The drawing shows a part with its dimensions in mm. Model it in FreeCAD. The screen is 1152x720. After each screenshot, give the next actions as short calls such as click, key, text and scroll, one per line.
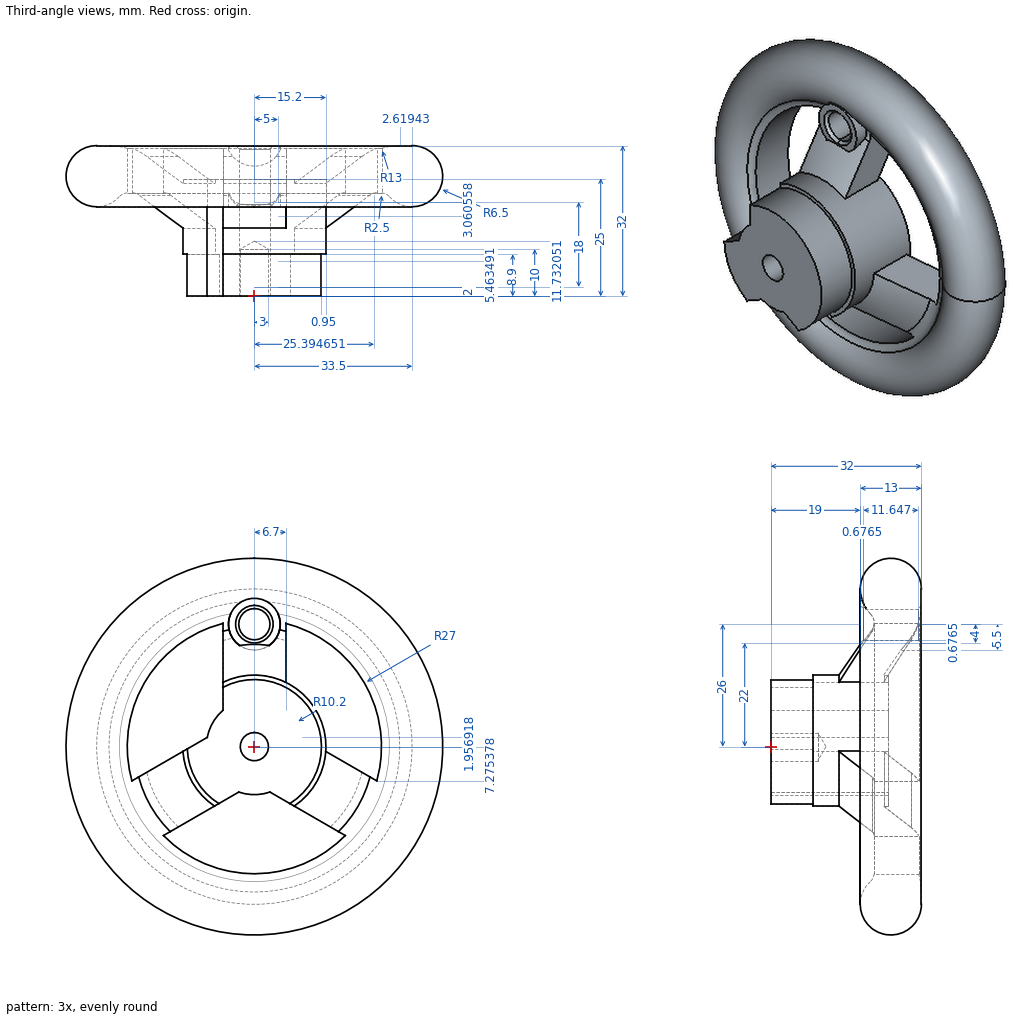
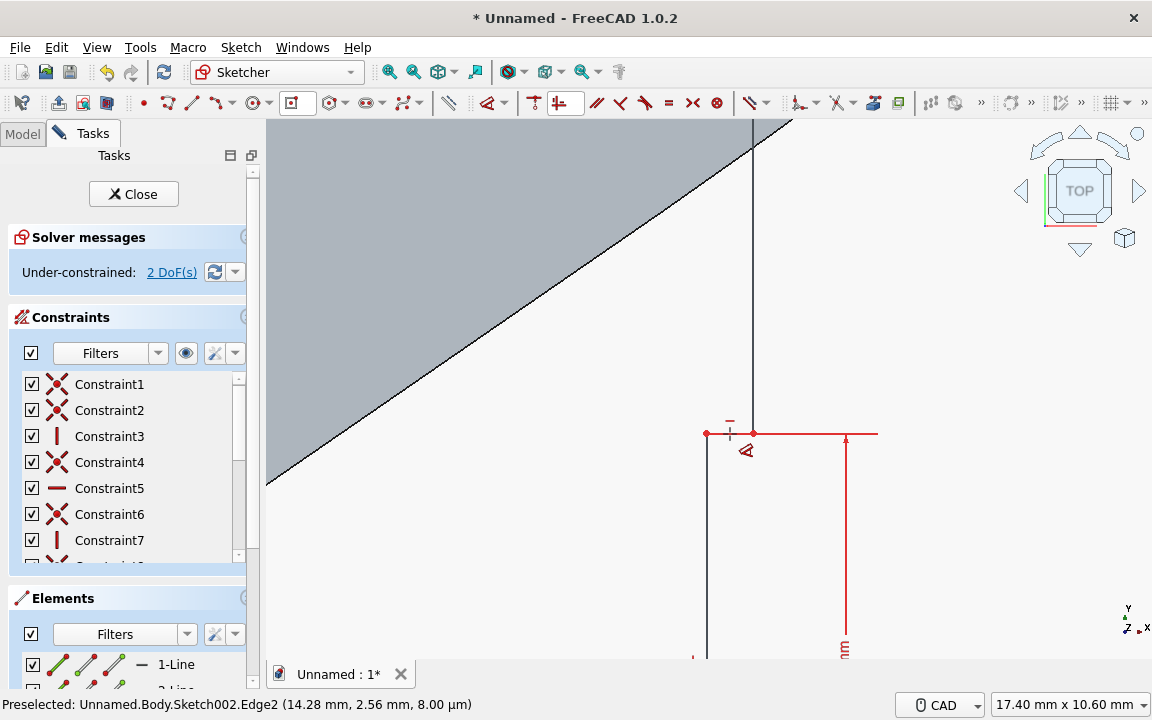
click(730, 434)
click(730, 468)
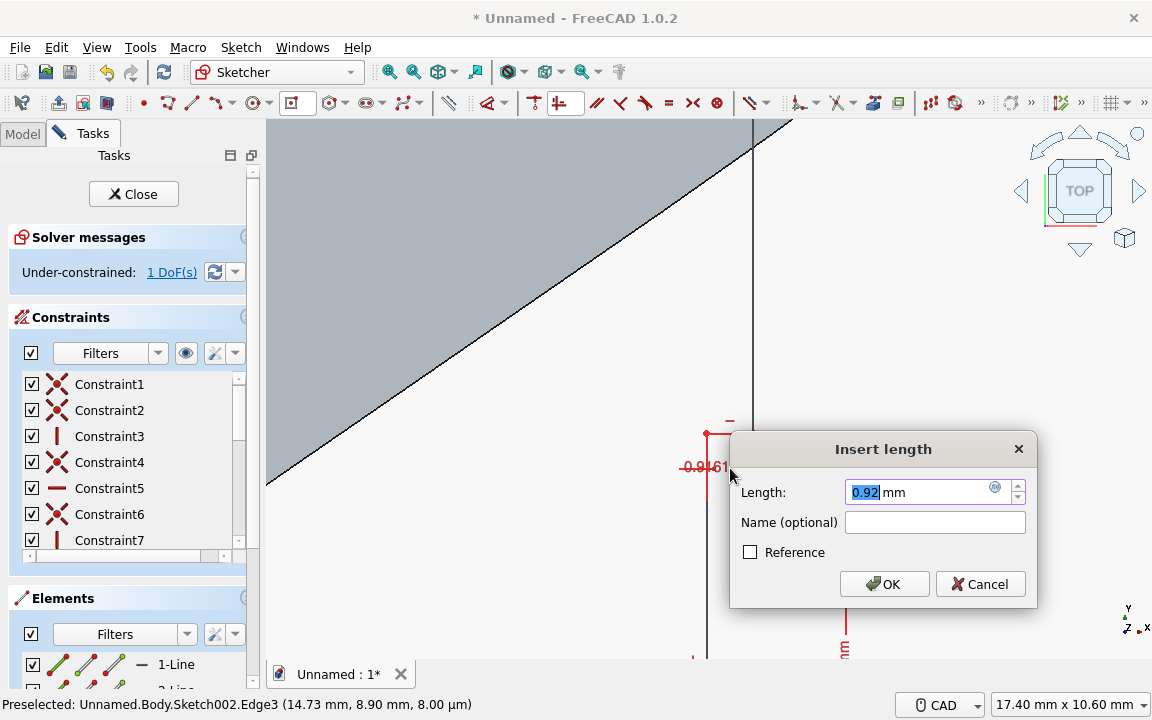
text(0.95)
key(Return)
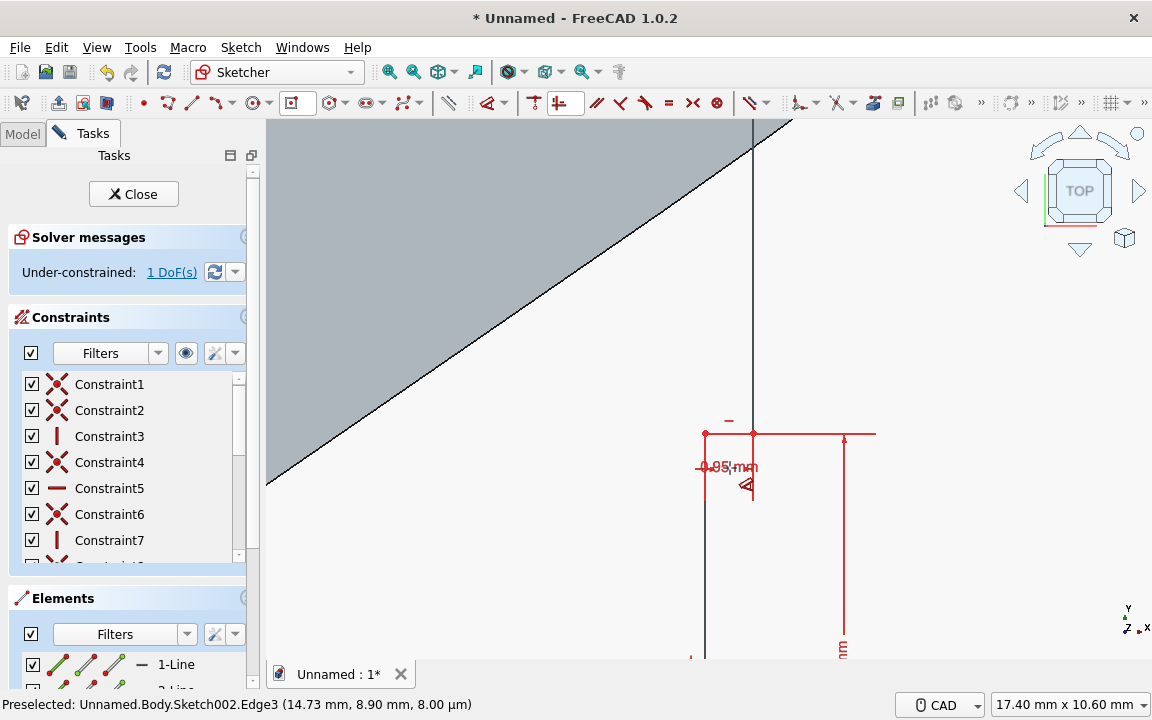
scroll(730, 434, down, 7)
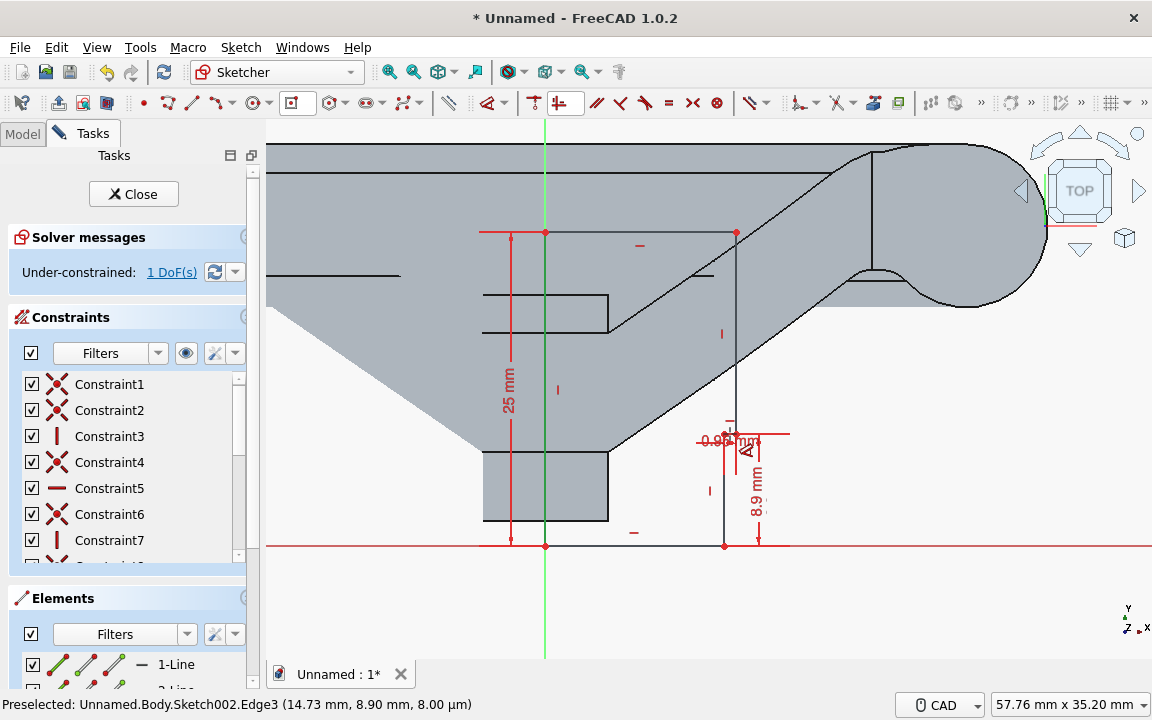
click(679, 232)
click(641, 198)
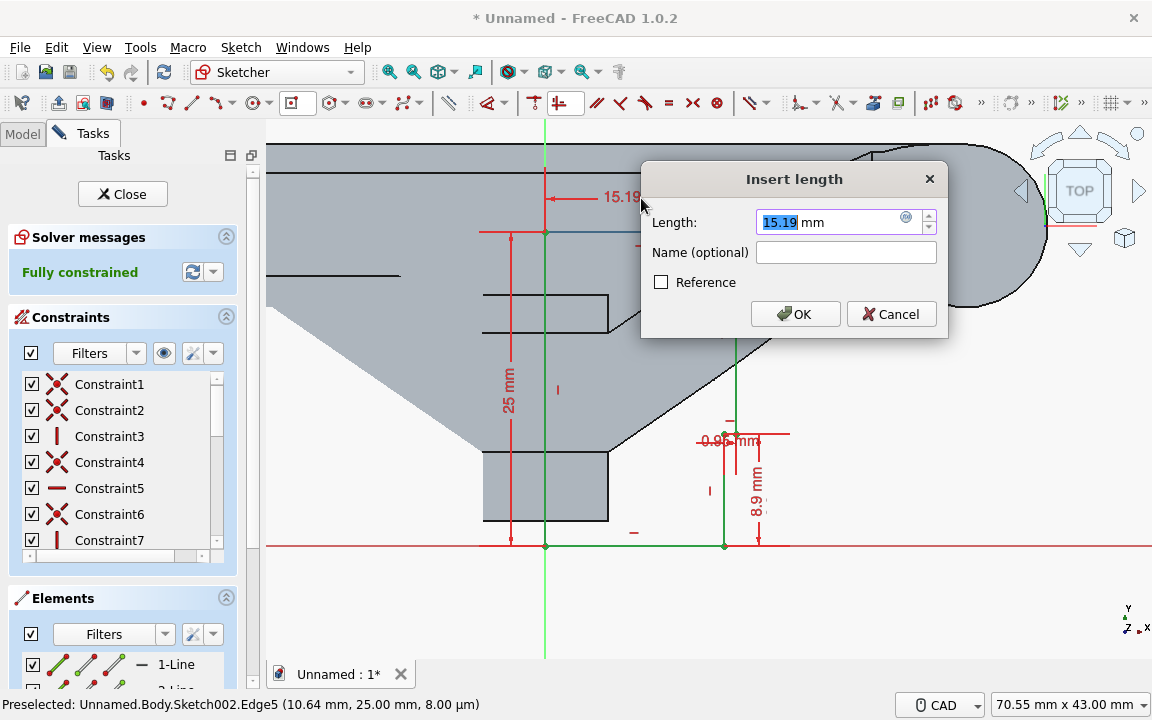
text(15.2)
key(Return)
key(Escape)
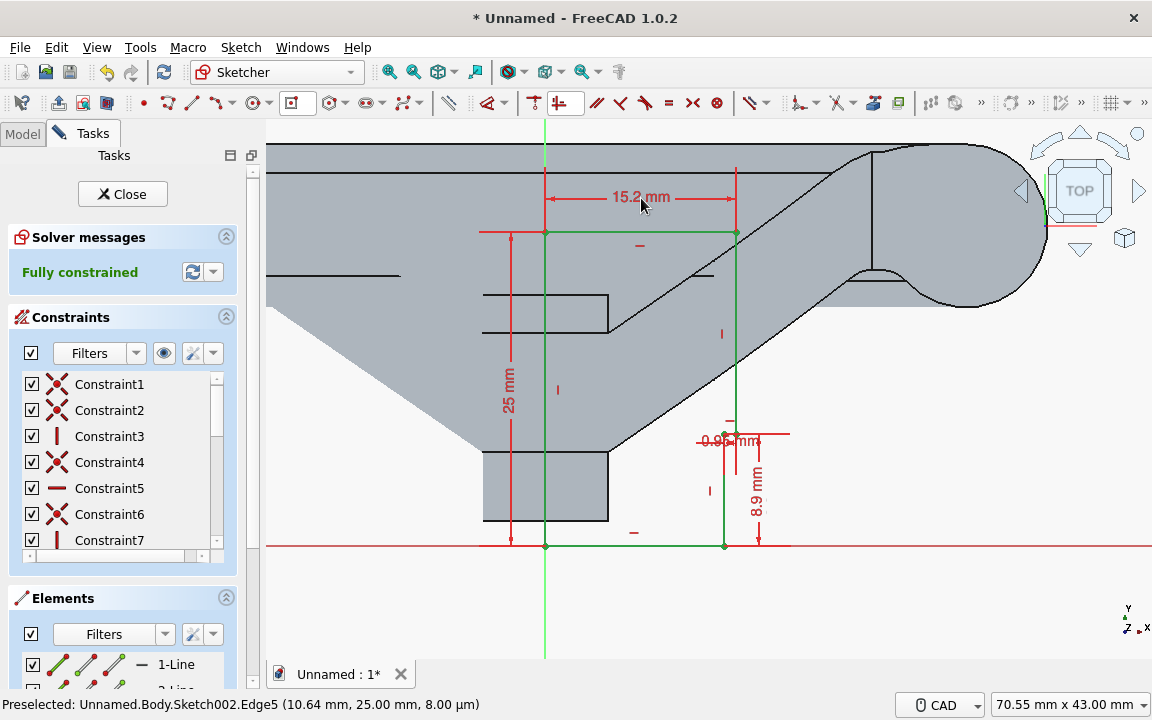
click(123, 194)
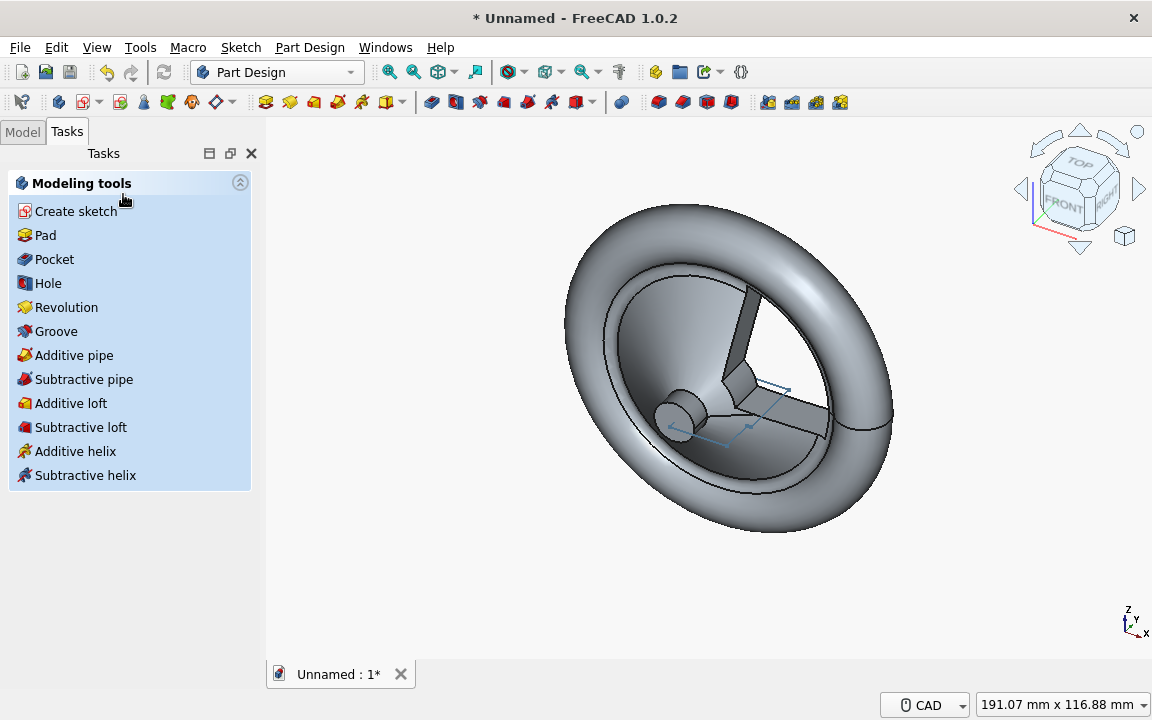
click(290, 102)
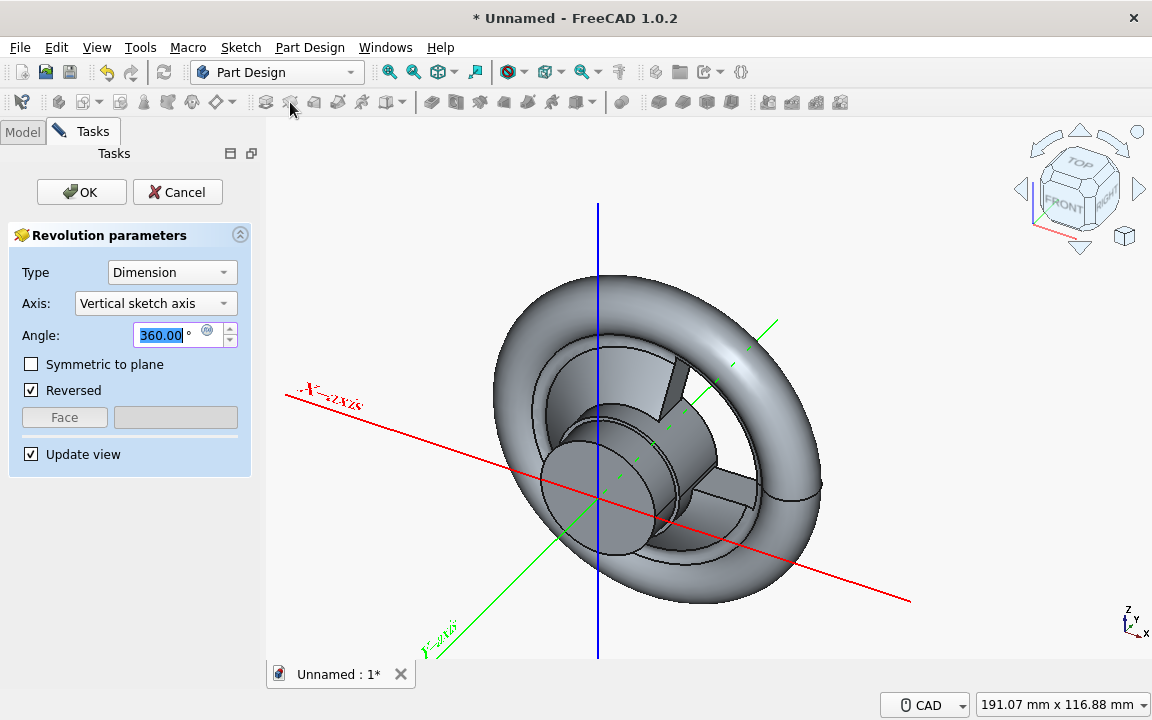
click(82, 192)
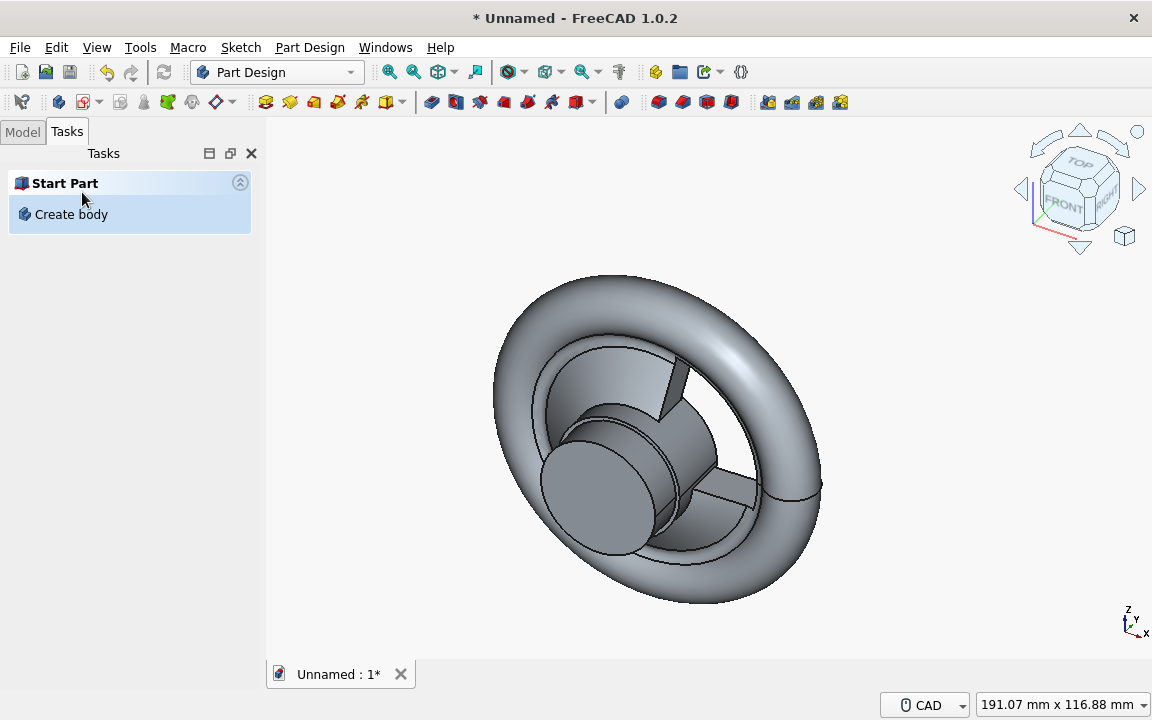
click(390, 72)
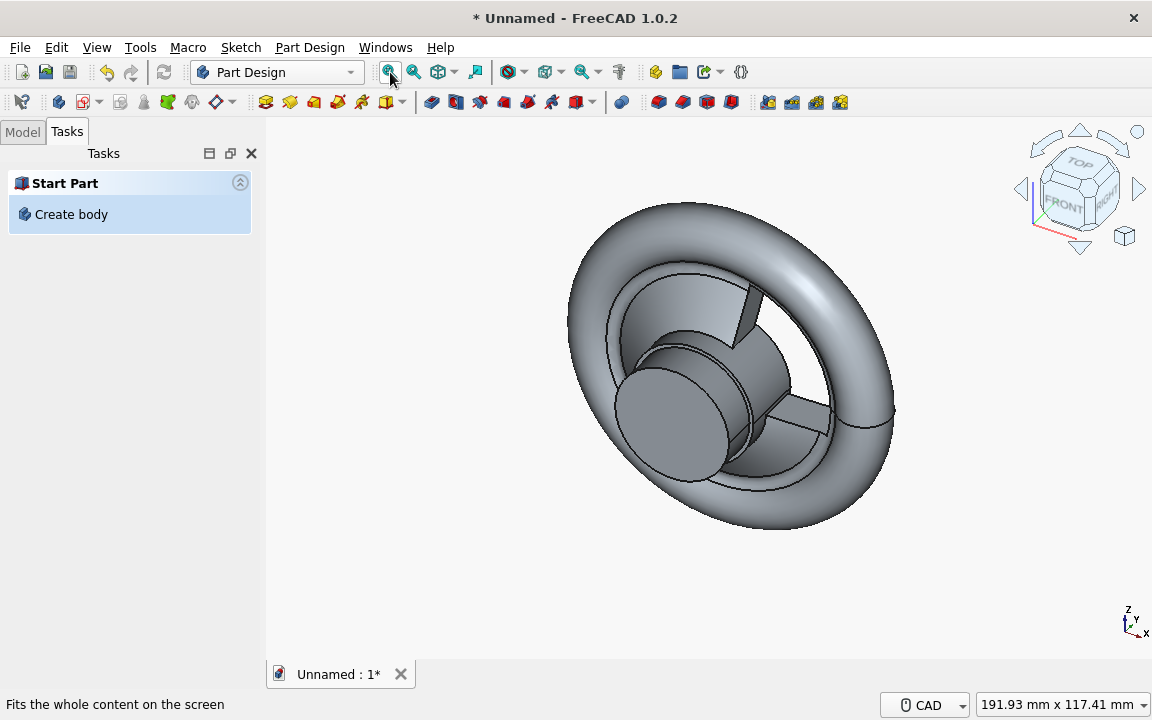
click(84, 102)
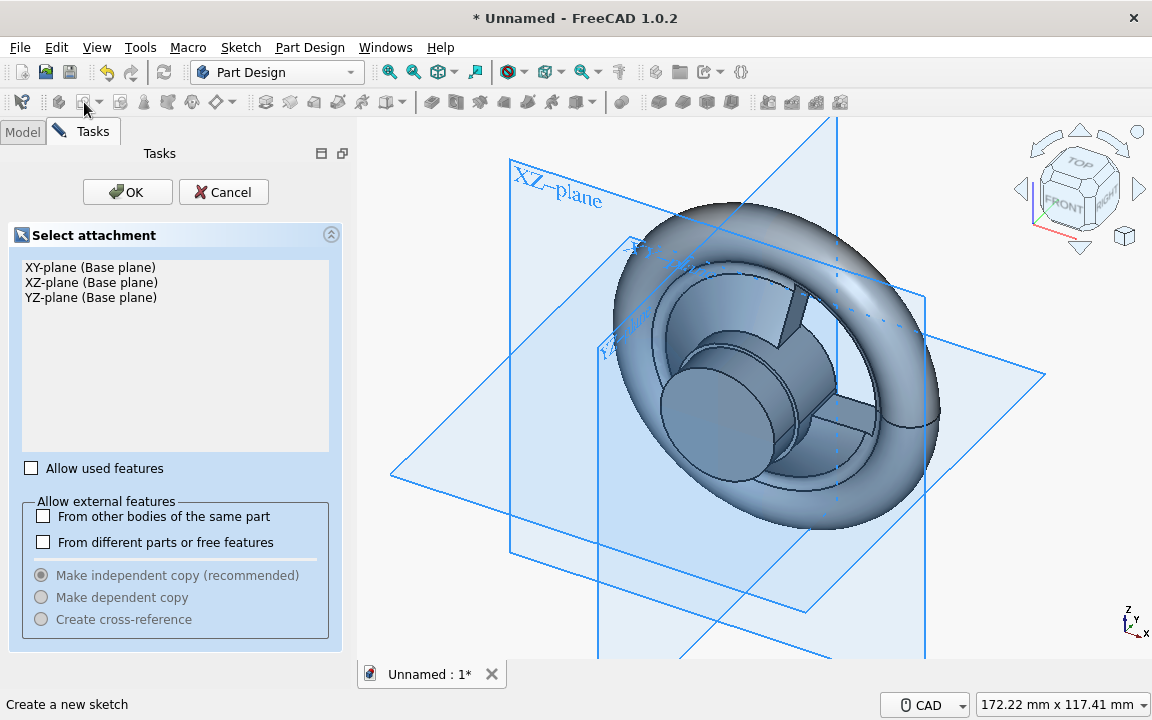
click(82, 298)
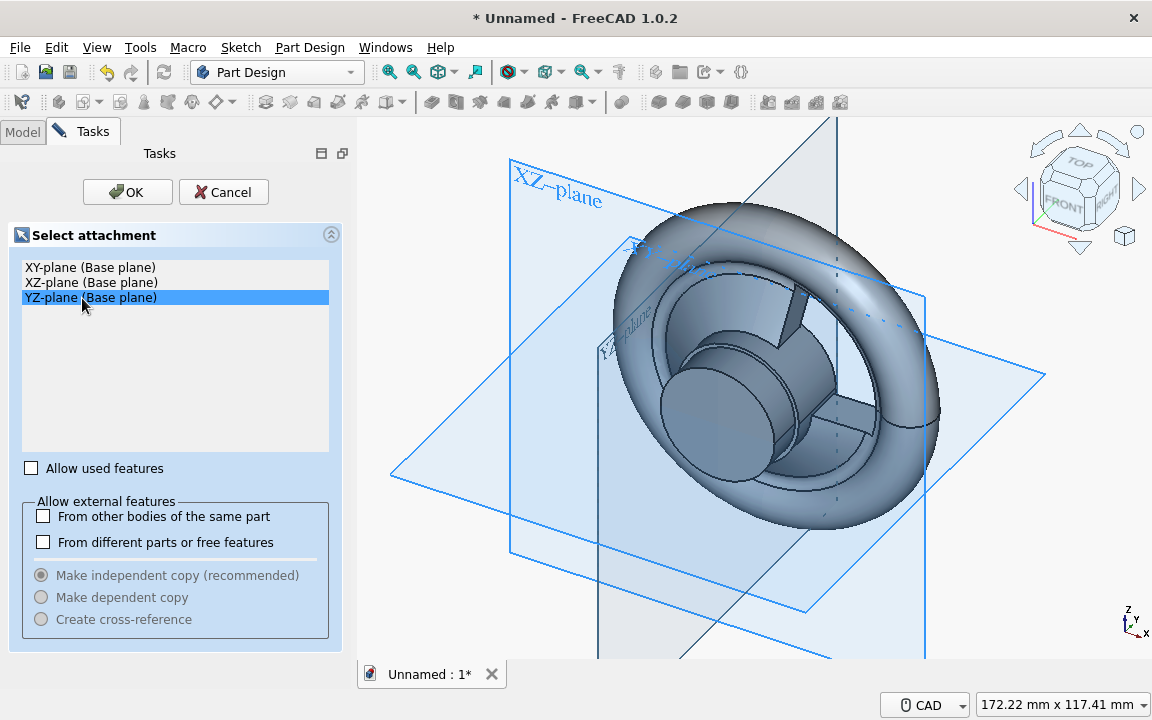
click(128, 192)